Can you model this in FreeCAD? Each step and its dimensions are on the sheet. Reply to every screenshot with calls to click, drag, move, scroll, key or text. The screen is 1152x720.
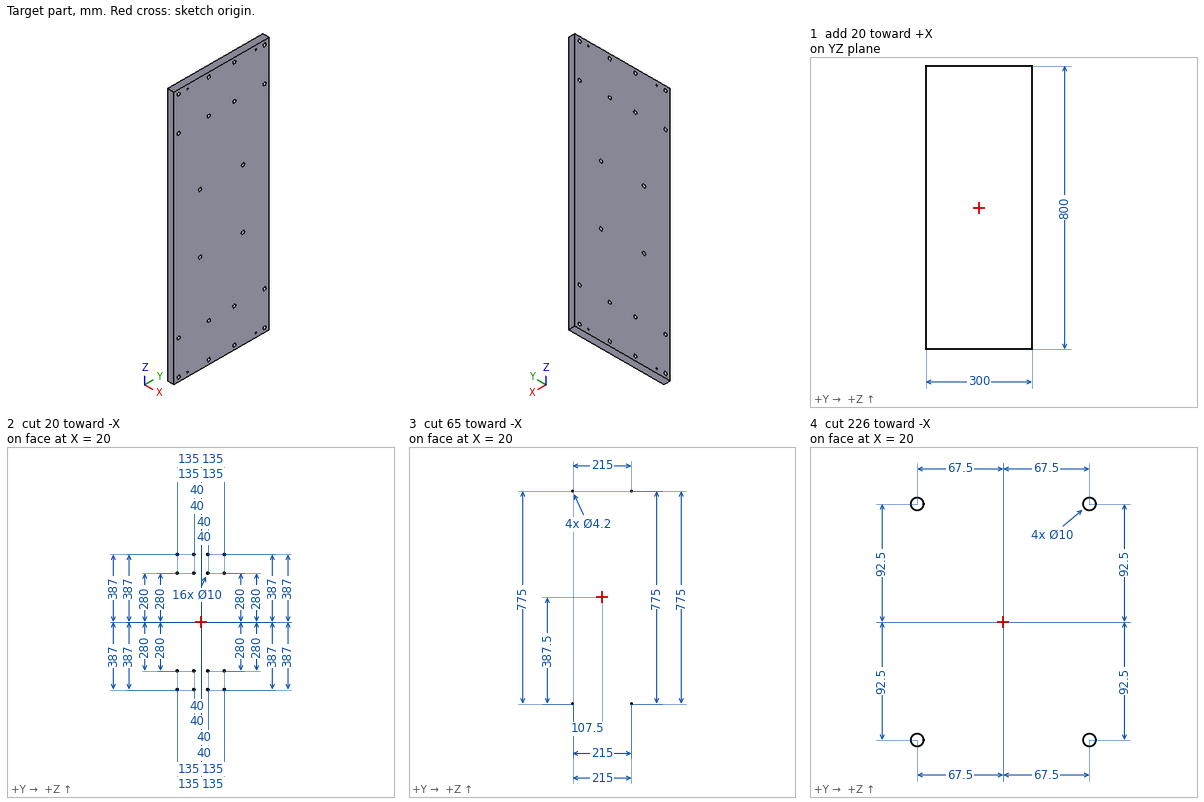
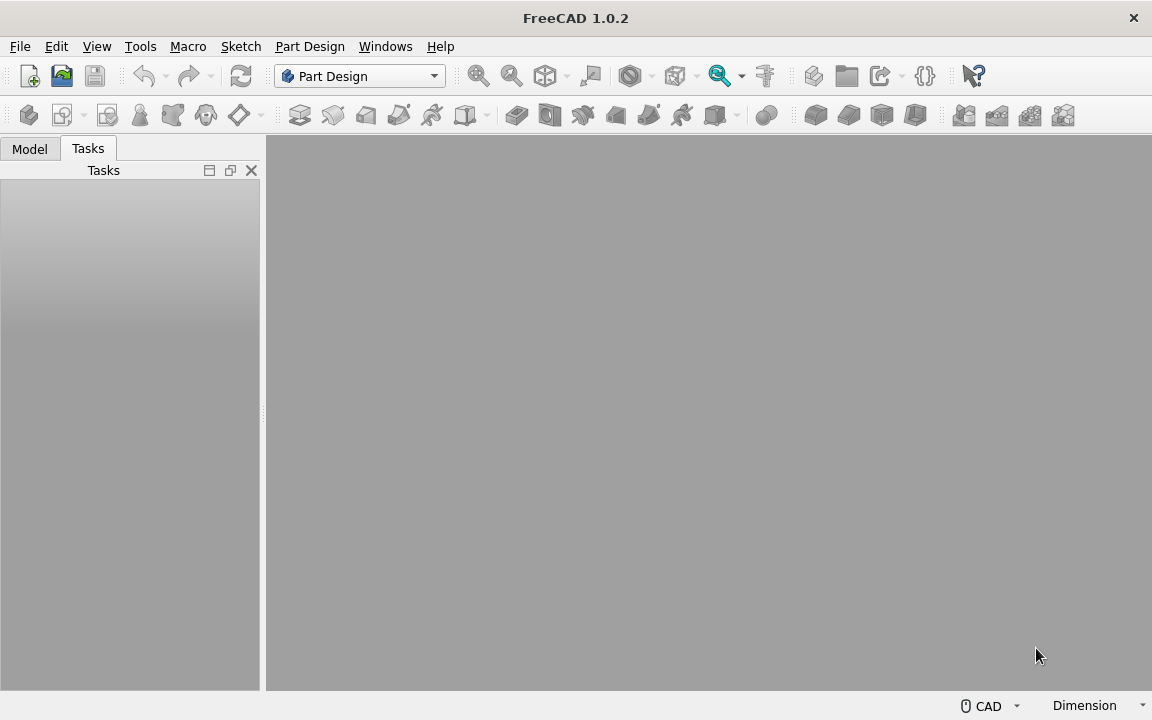
key(ctrl+n)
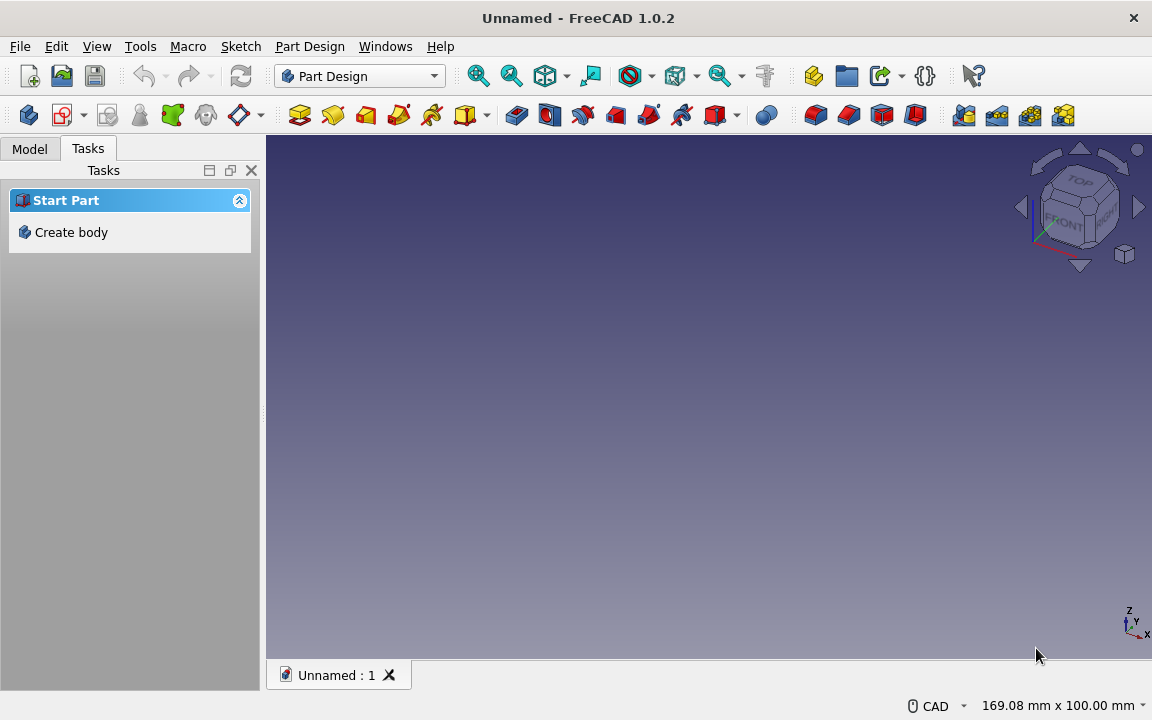
click(62, 116)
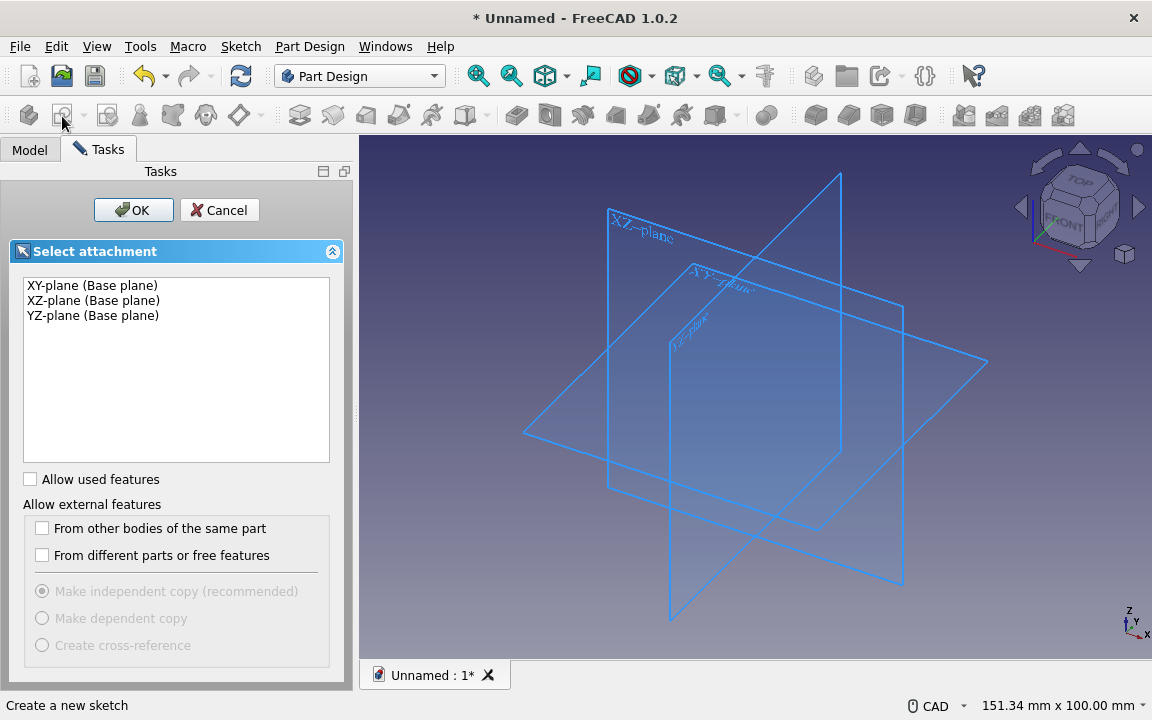
click(84, 316)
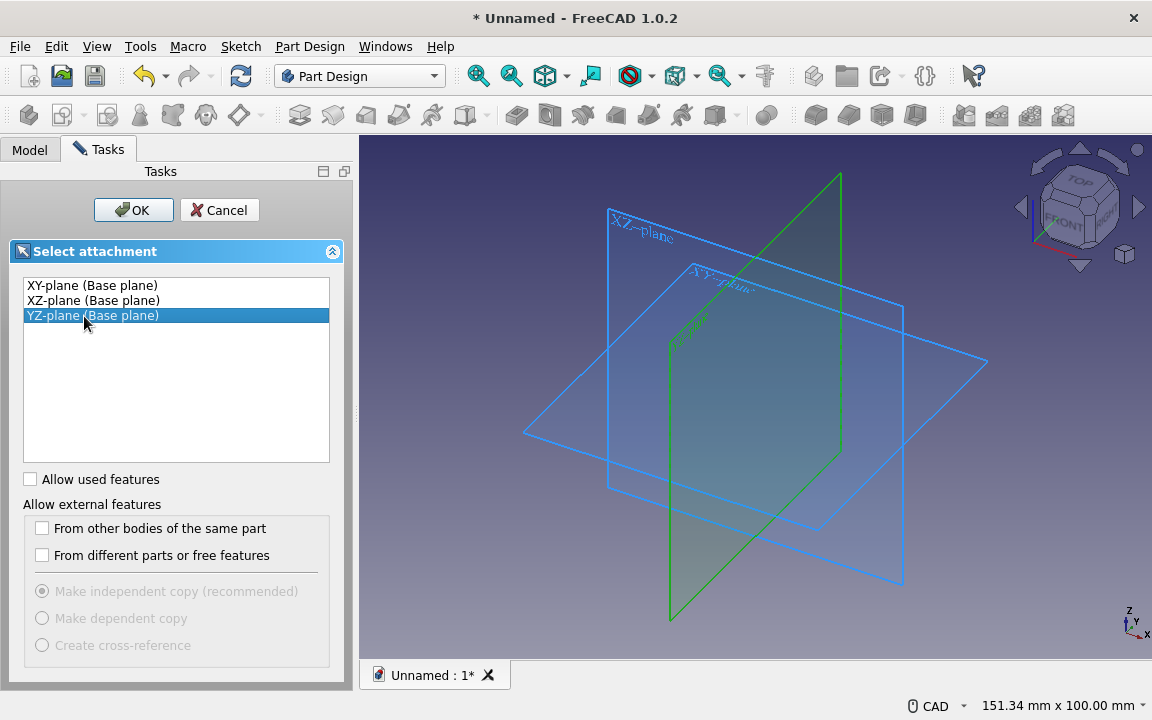
click(134, 210)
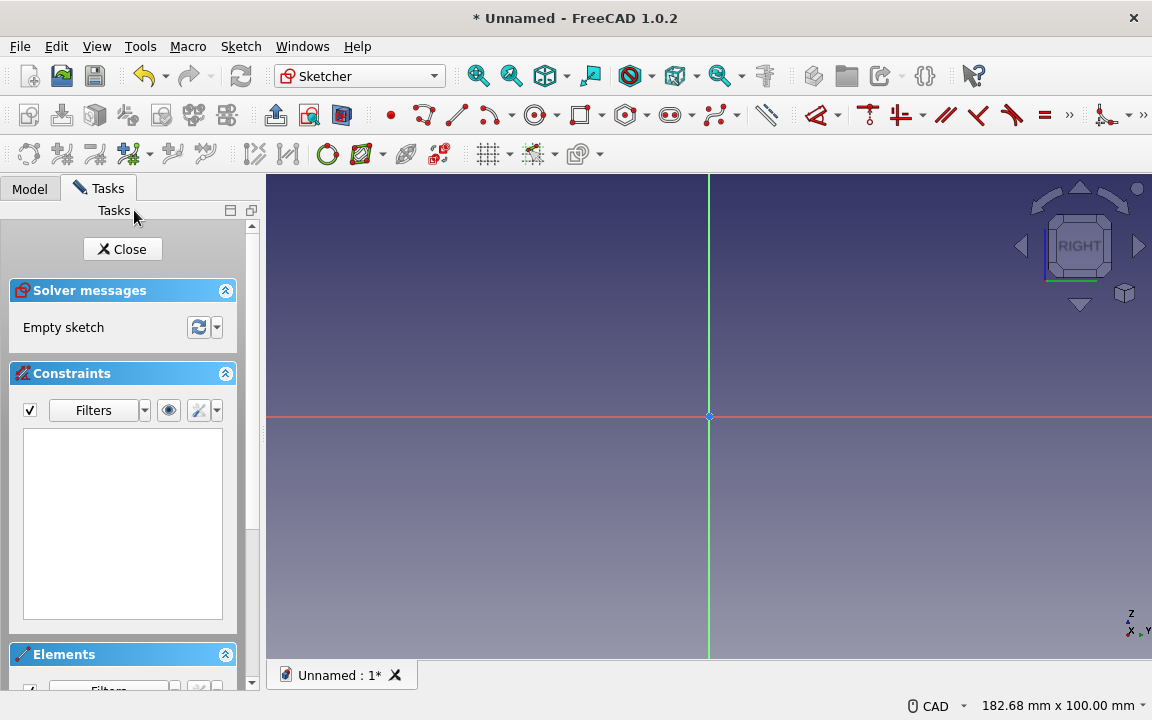
scroll(635, 416, down, 13)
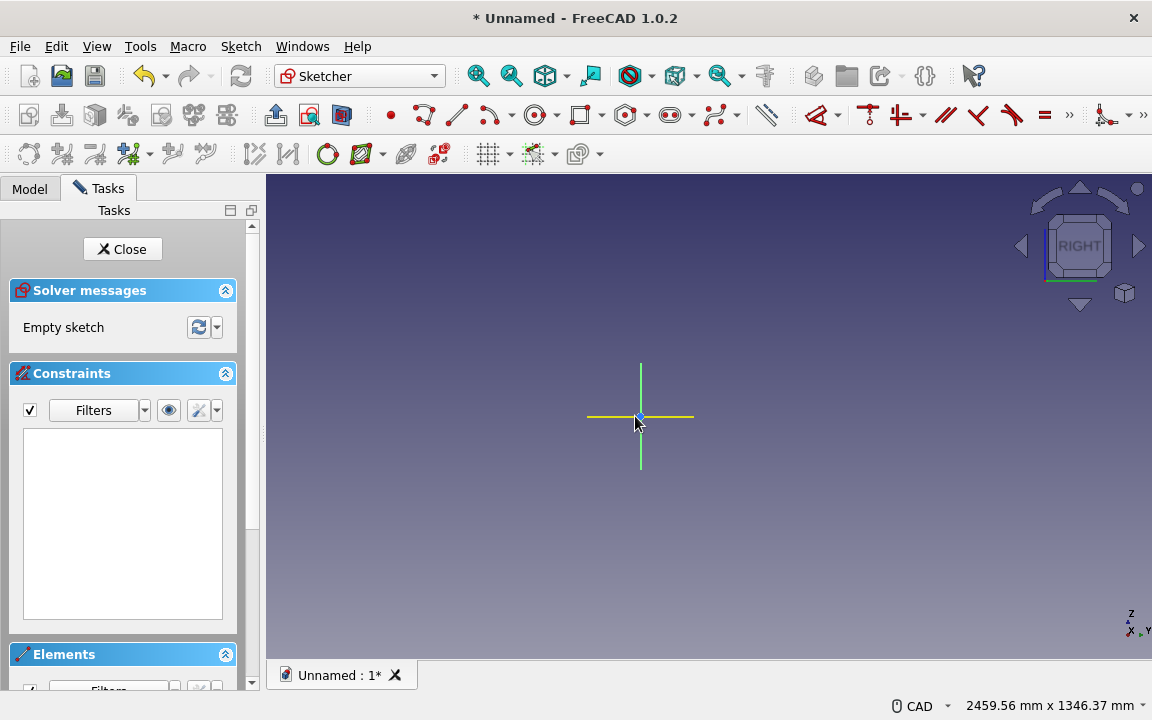
click(602, 116)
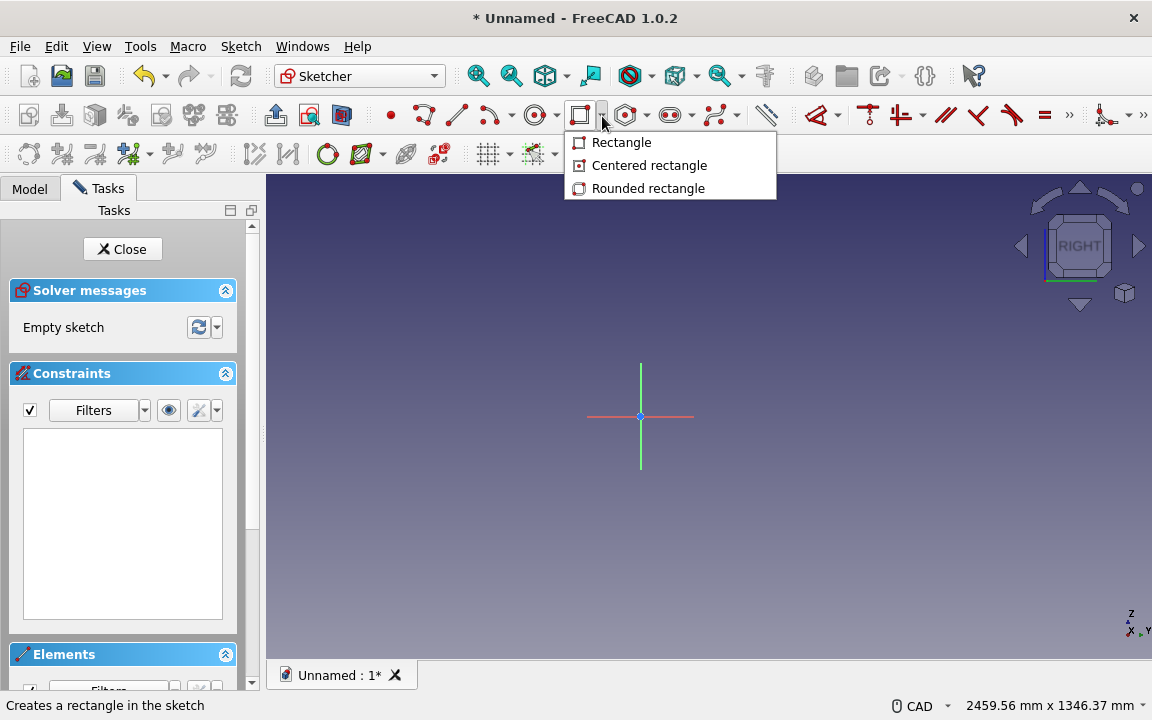
click(670, 166)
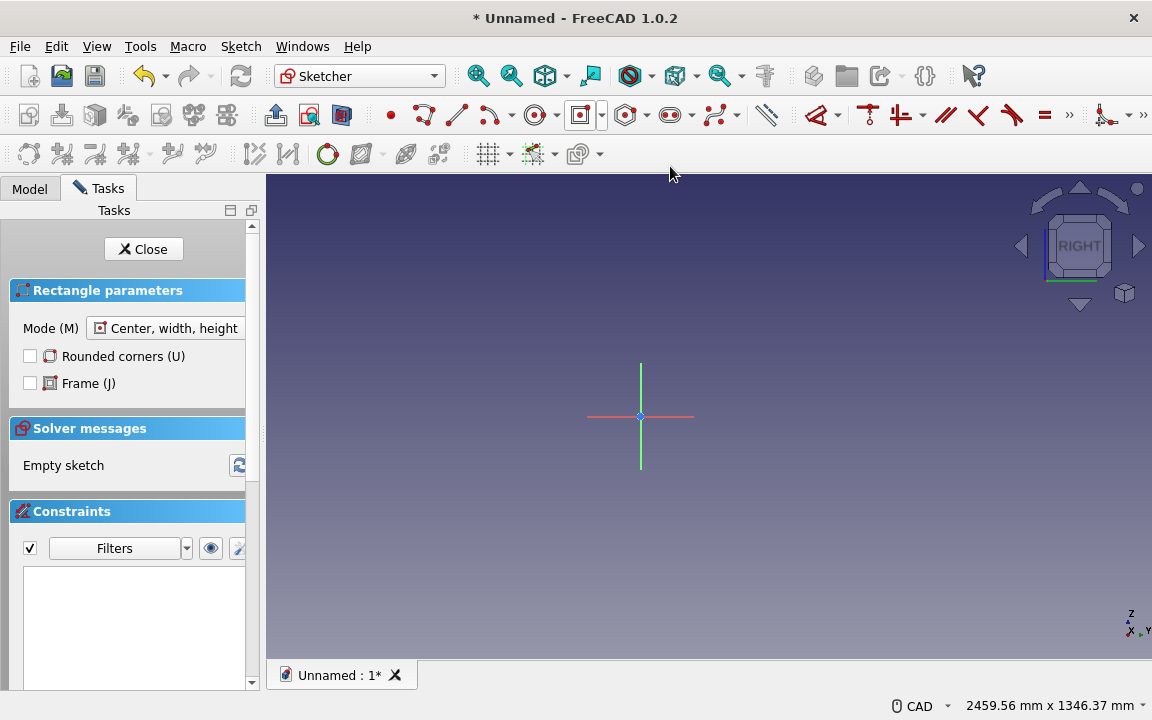
click(641, 416)
move(695, 272)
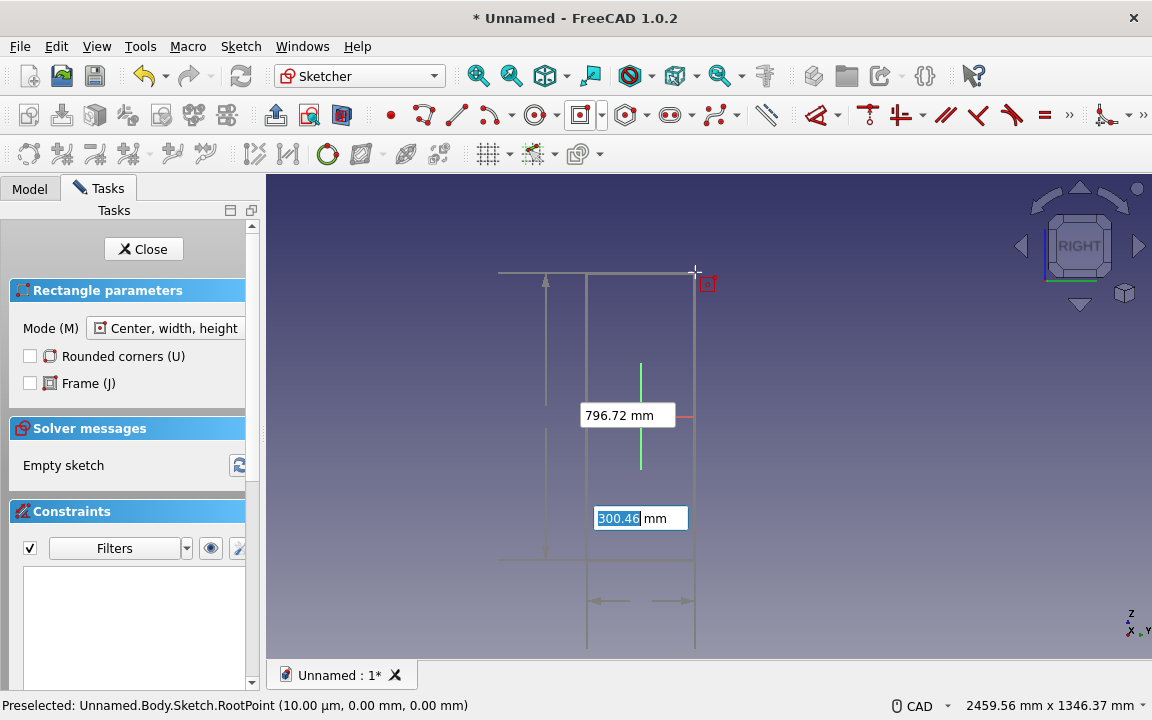
text(300)
key(Tab)
text(800)
key(Return)
key(Escape)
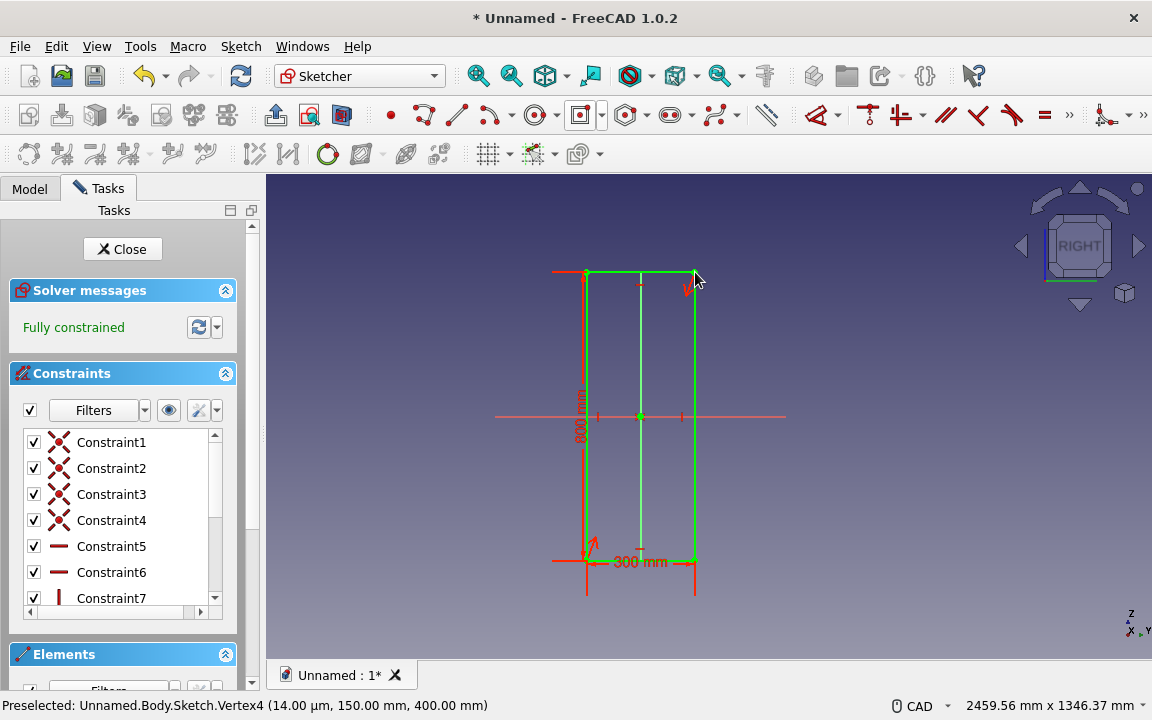
click(123, 249)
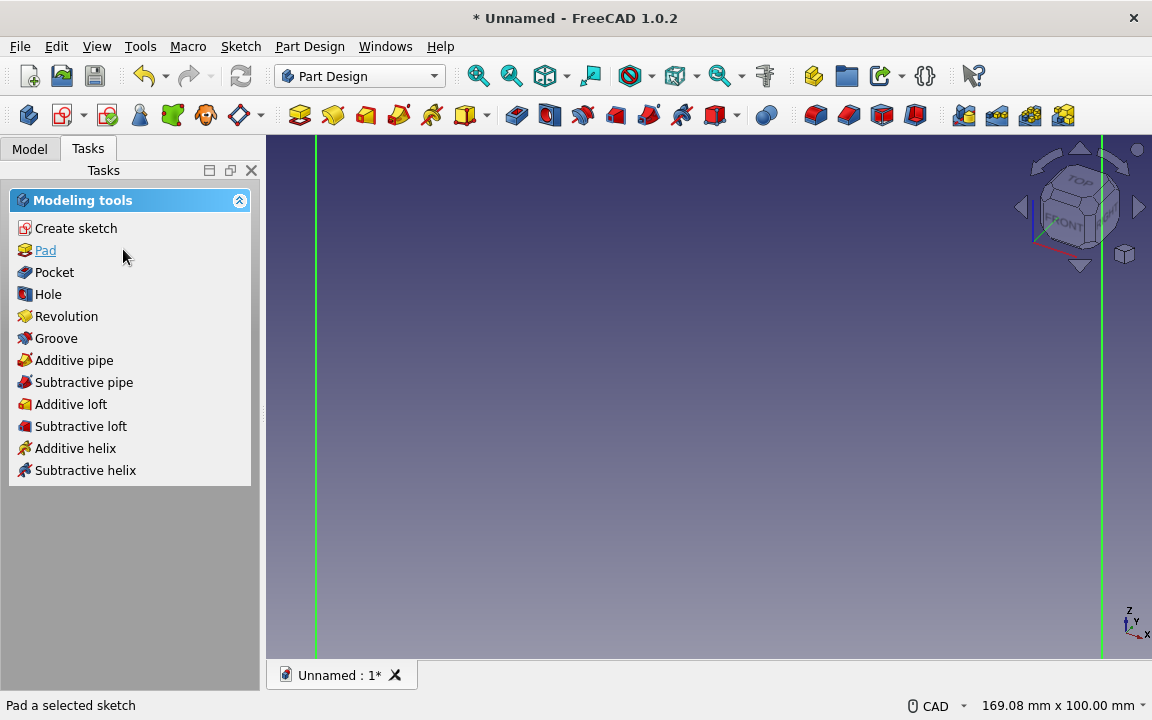
click(300, 116)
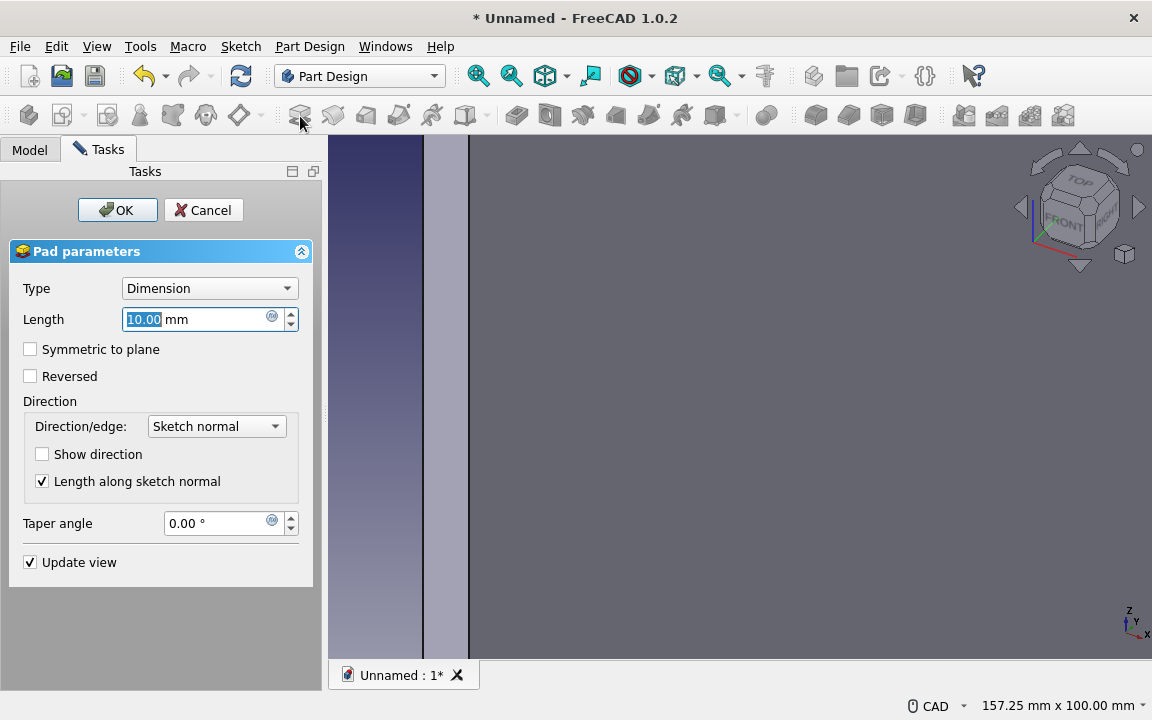
text(20)
key(Tab)